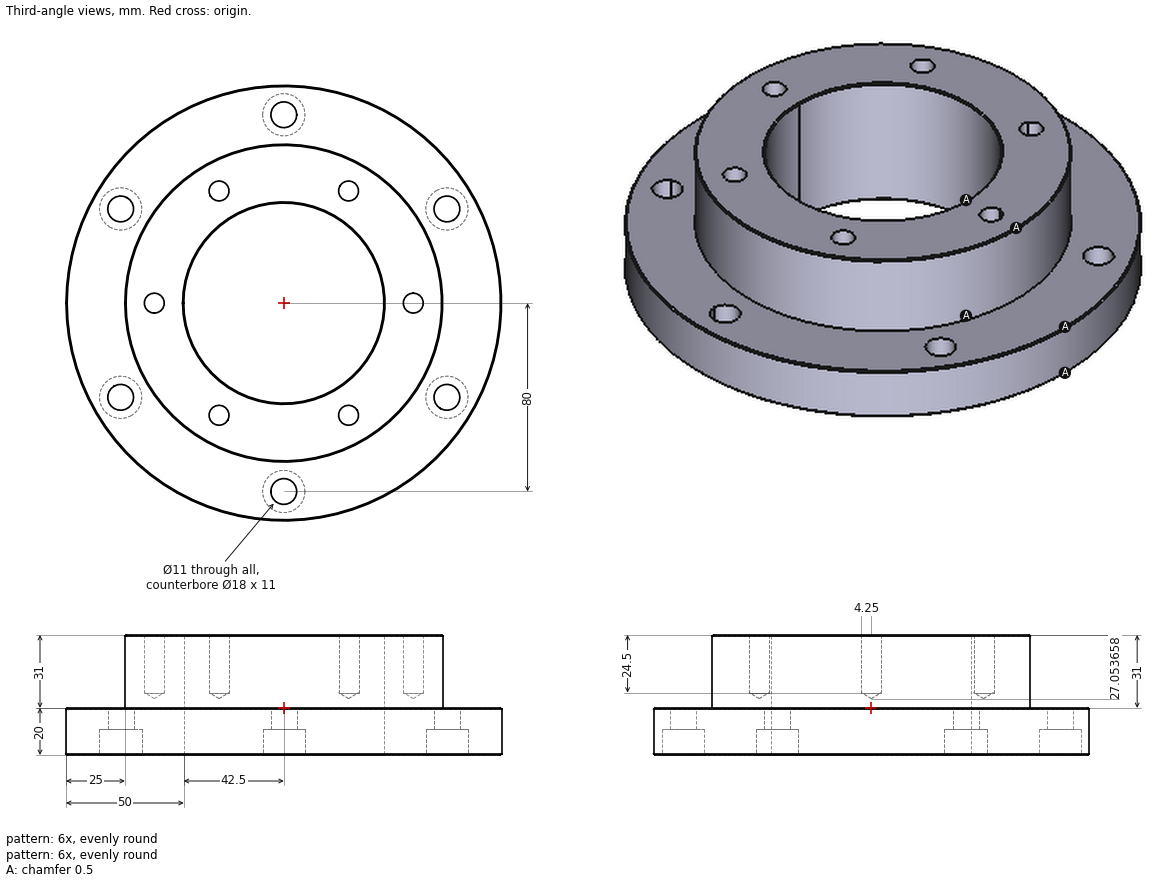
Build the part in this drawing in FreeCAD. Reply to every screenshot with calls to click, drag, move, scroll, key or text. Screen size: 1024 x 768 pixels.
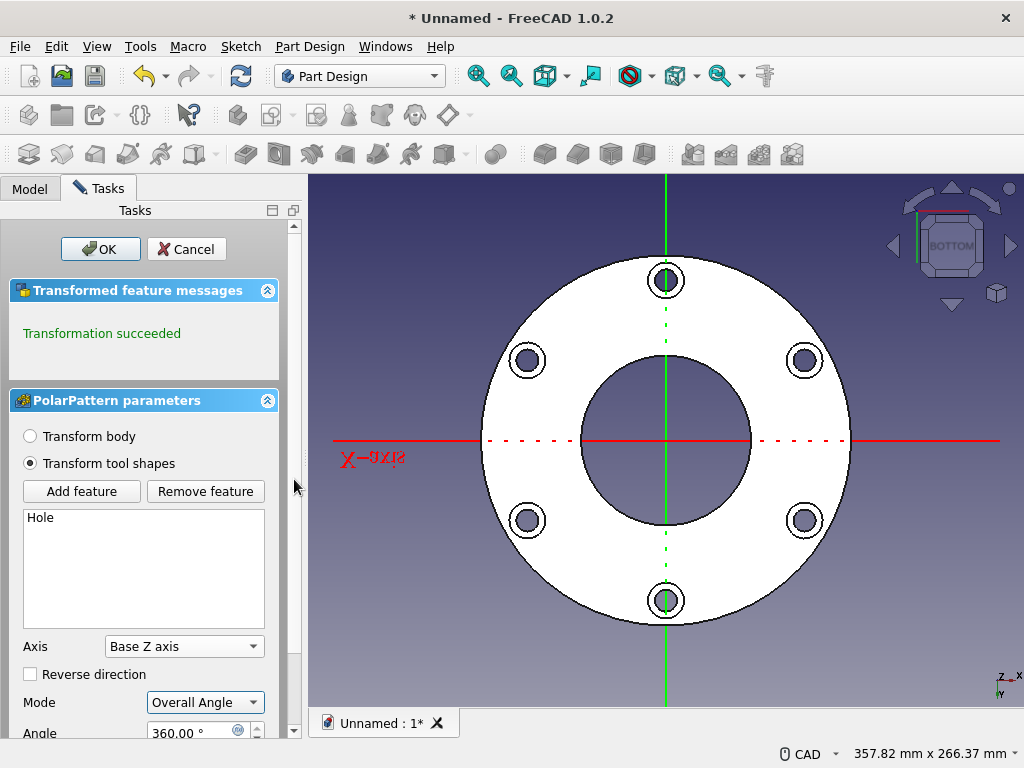
click(101, 249)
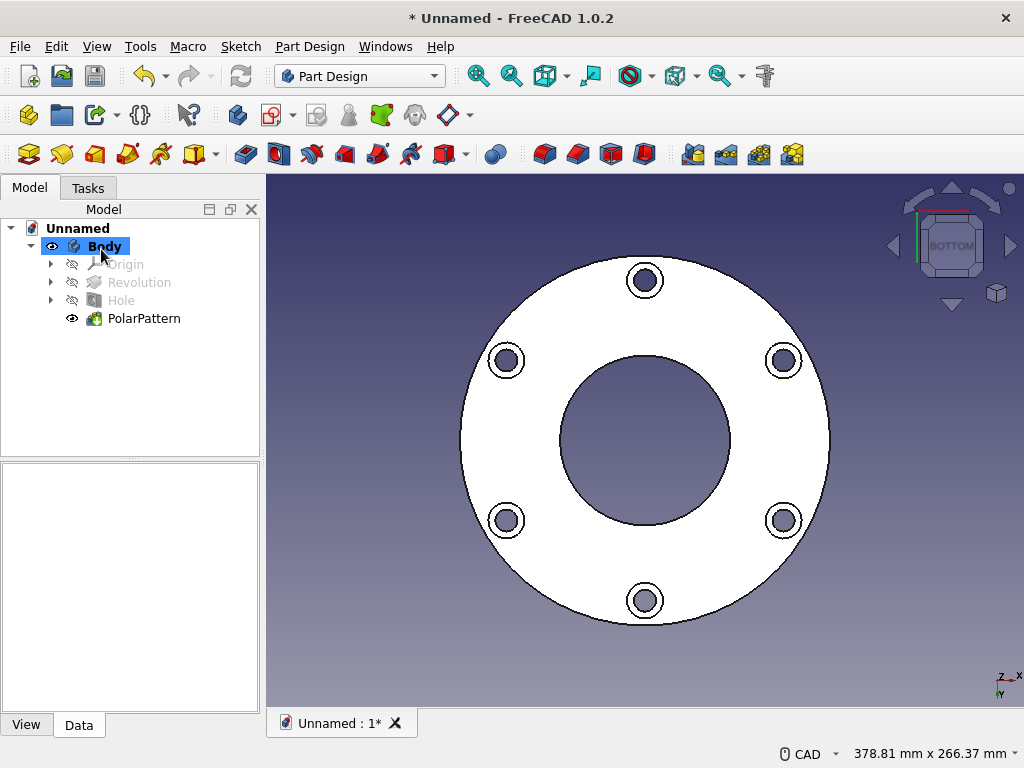
click(51, 264)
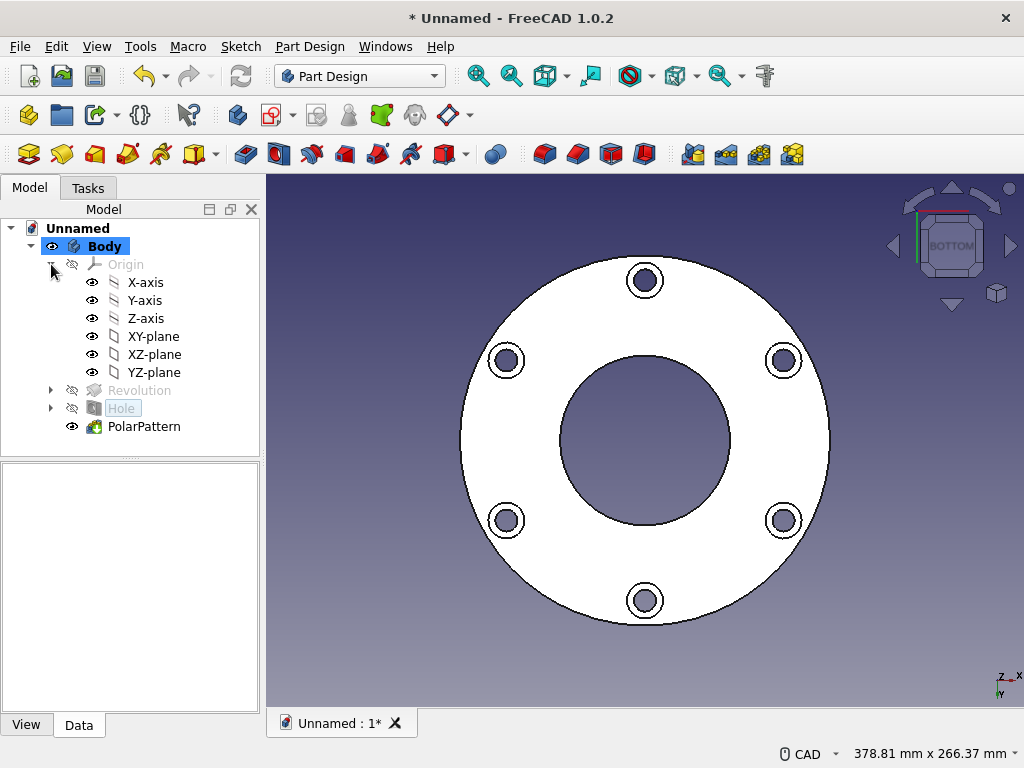
click(137, 372)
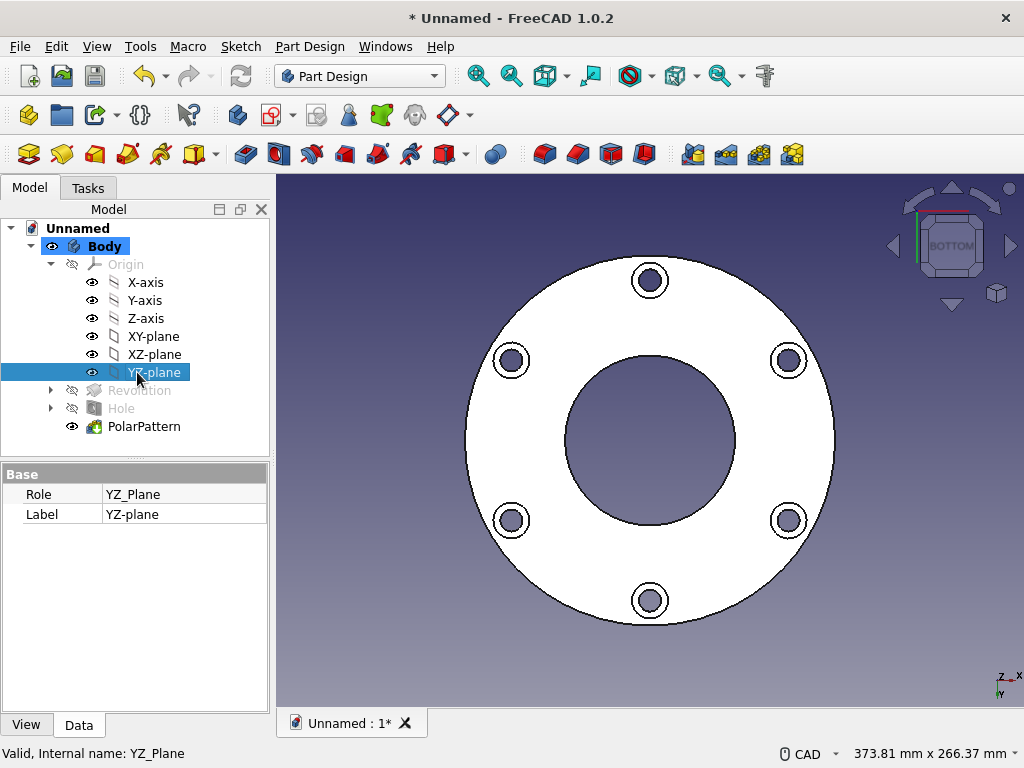
click(448, 116)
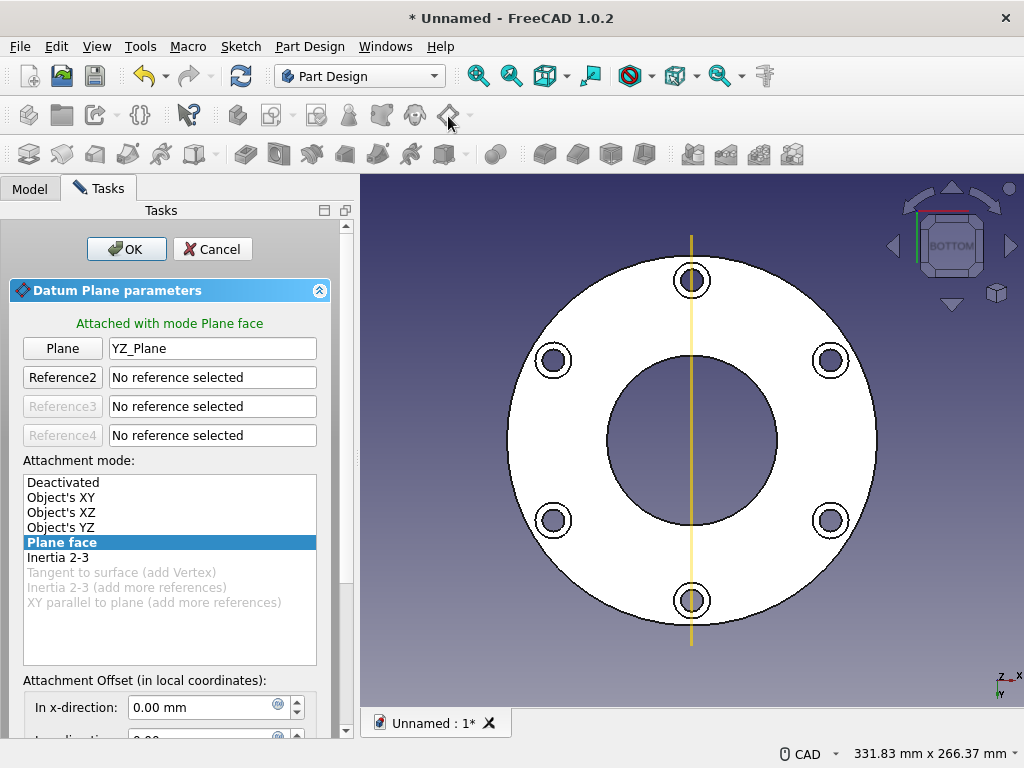
scroll(346, 479, down, 2)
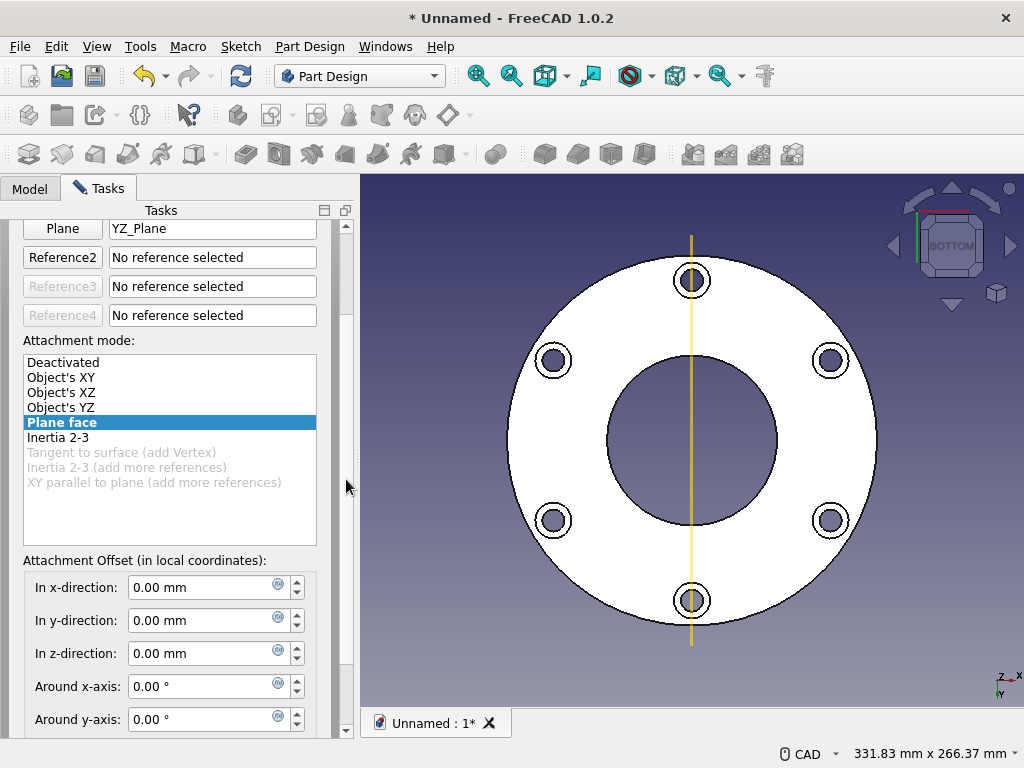
triple_click(210, 654)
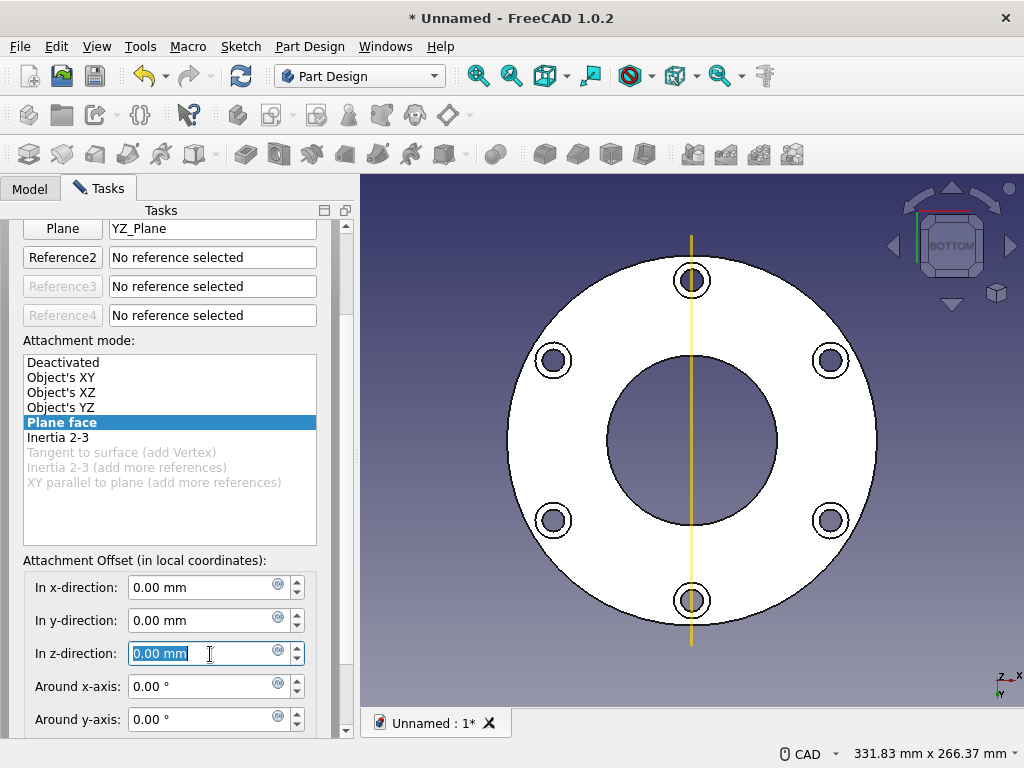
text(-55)
key(Tab)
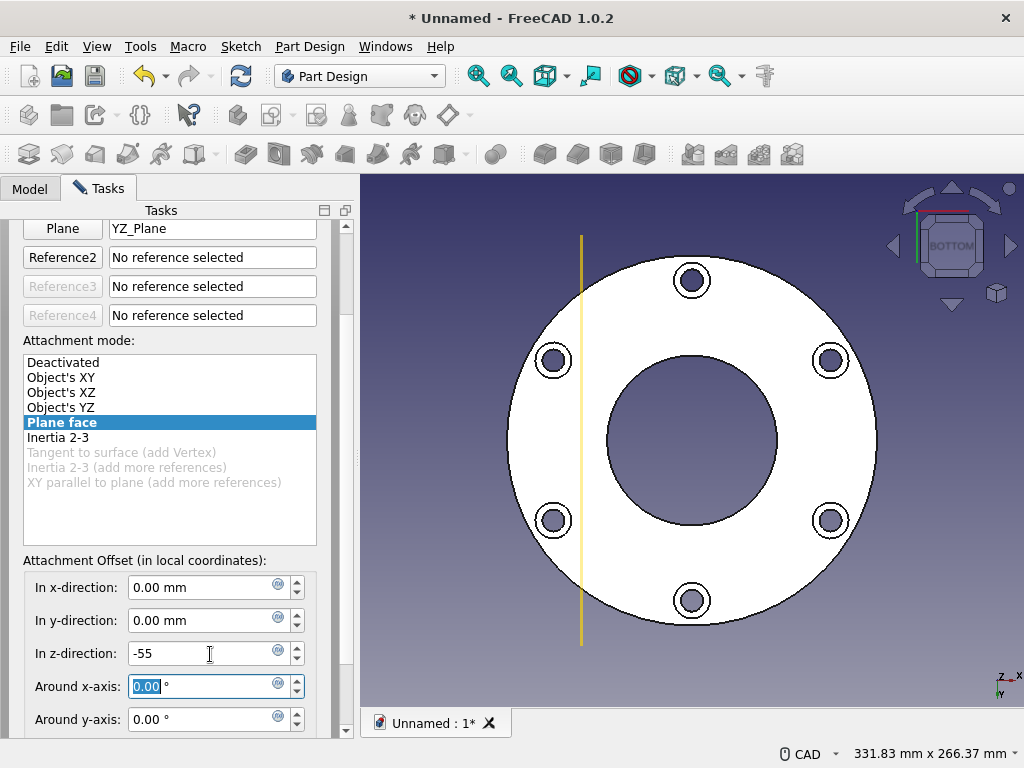
scroll(346, 479, up, 3)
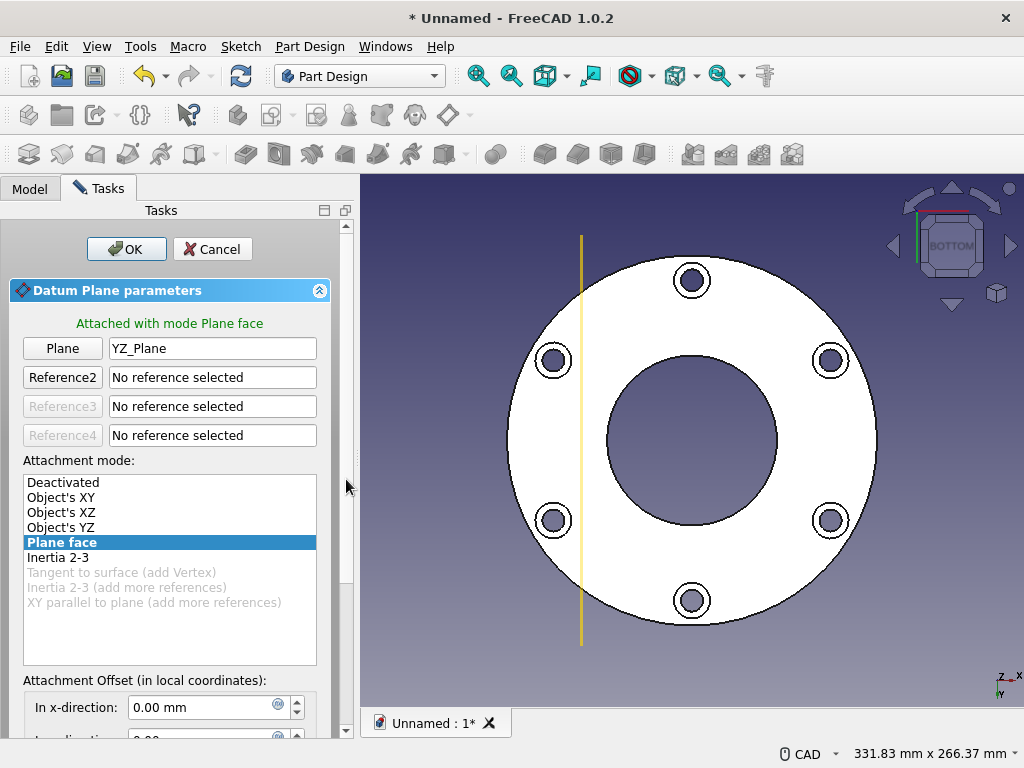
click(127, 249)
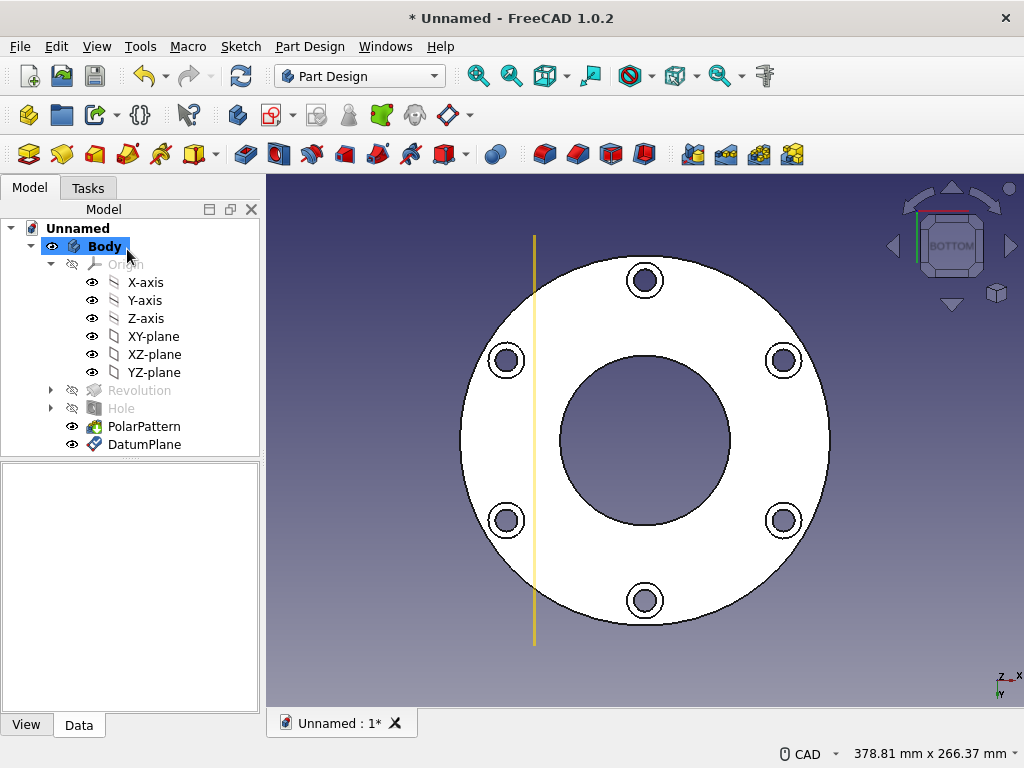
click(117, 444)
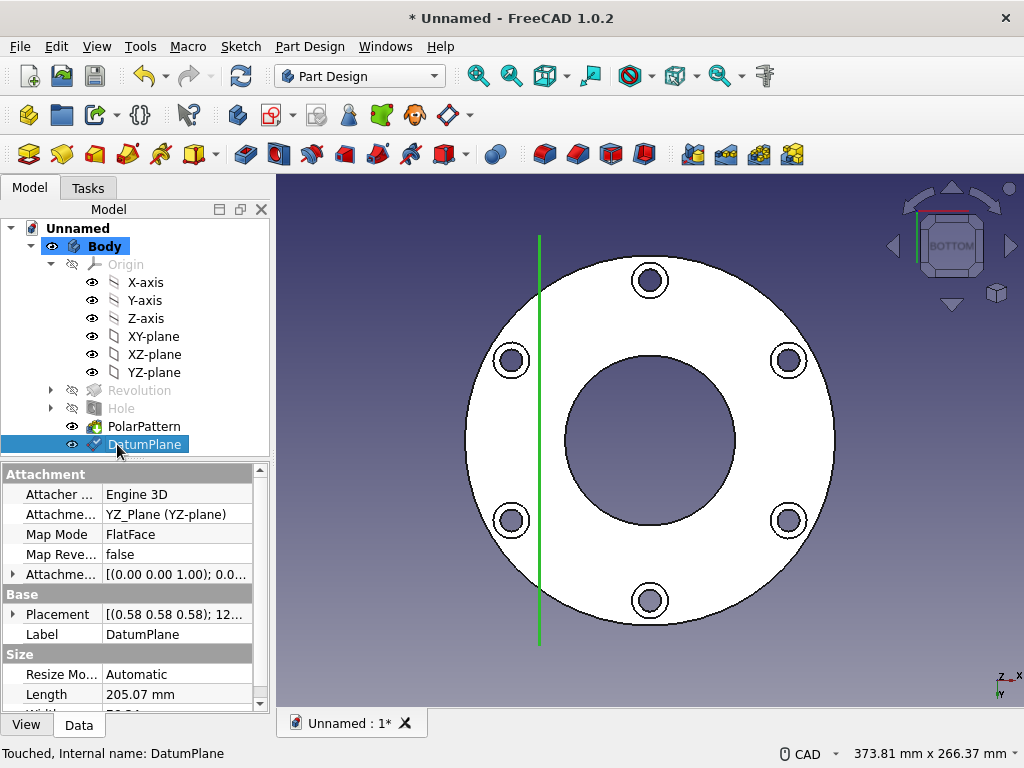
click(270, 116)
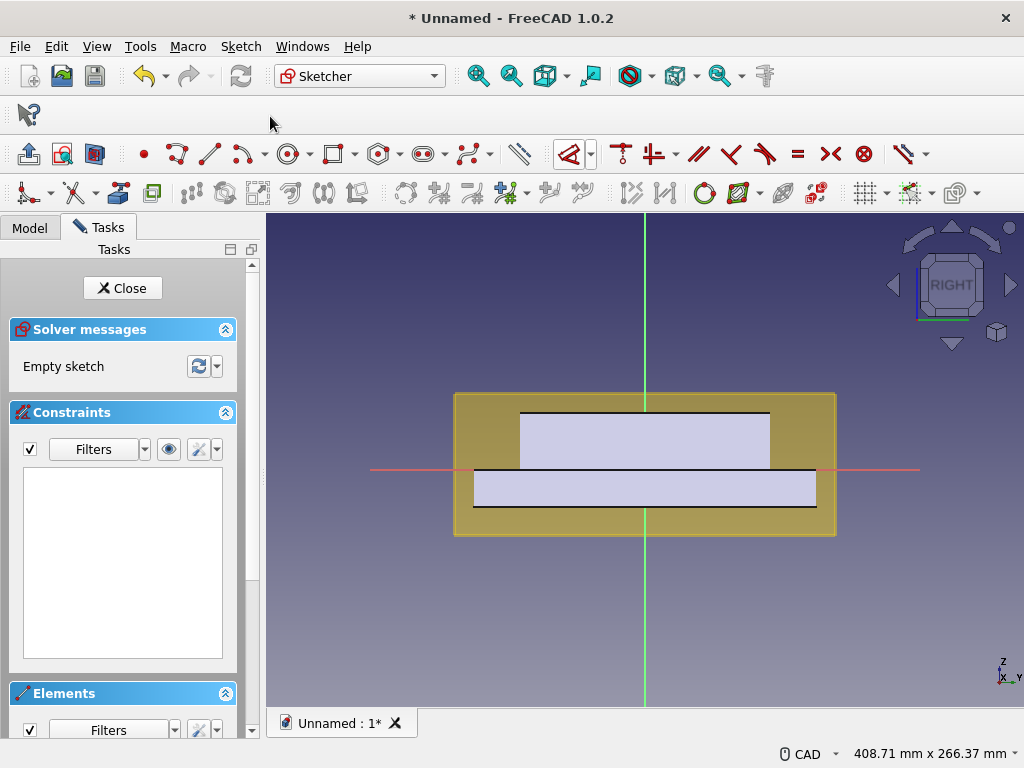
click(95, 154)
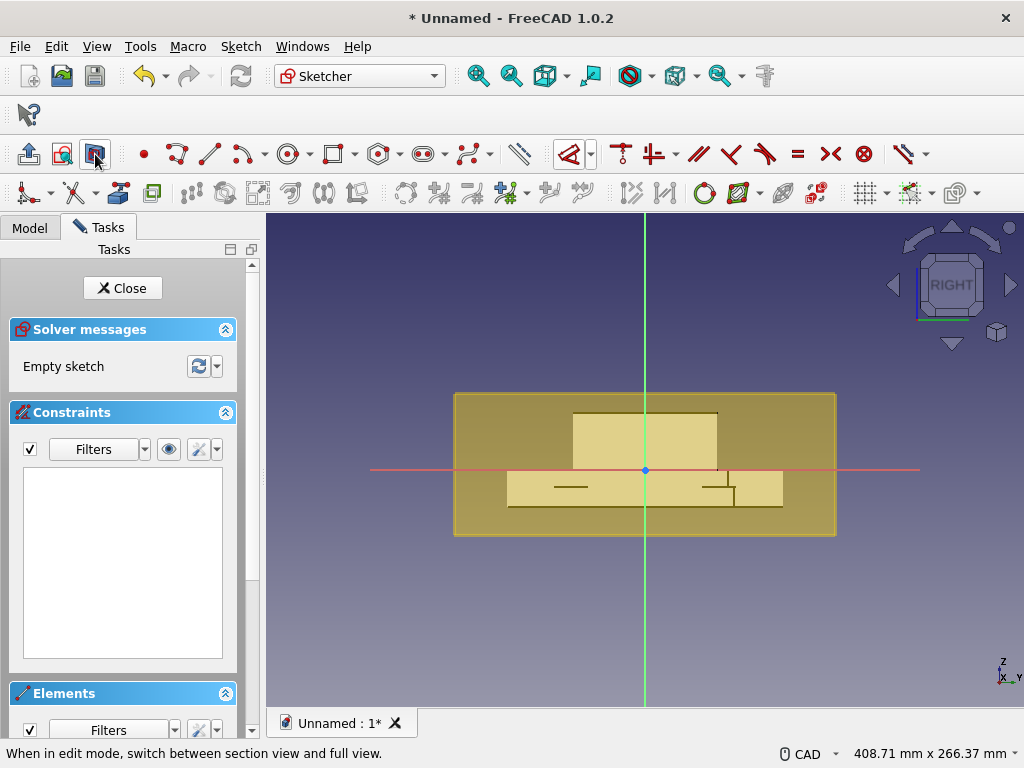
scroll(657, 437, up, 8)